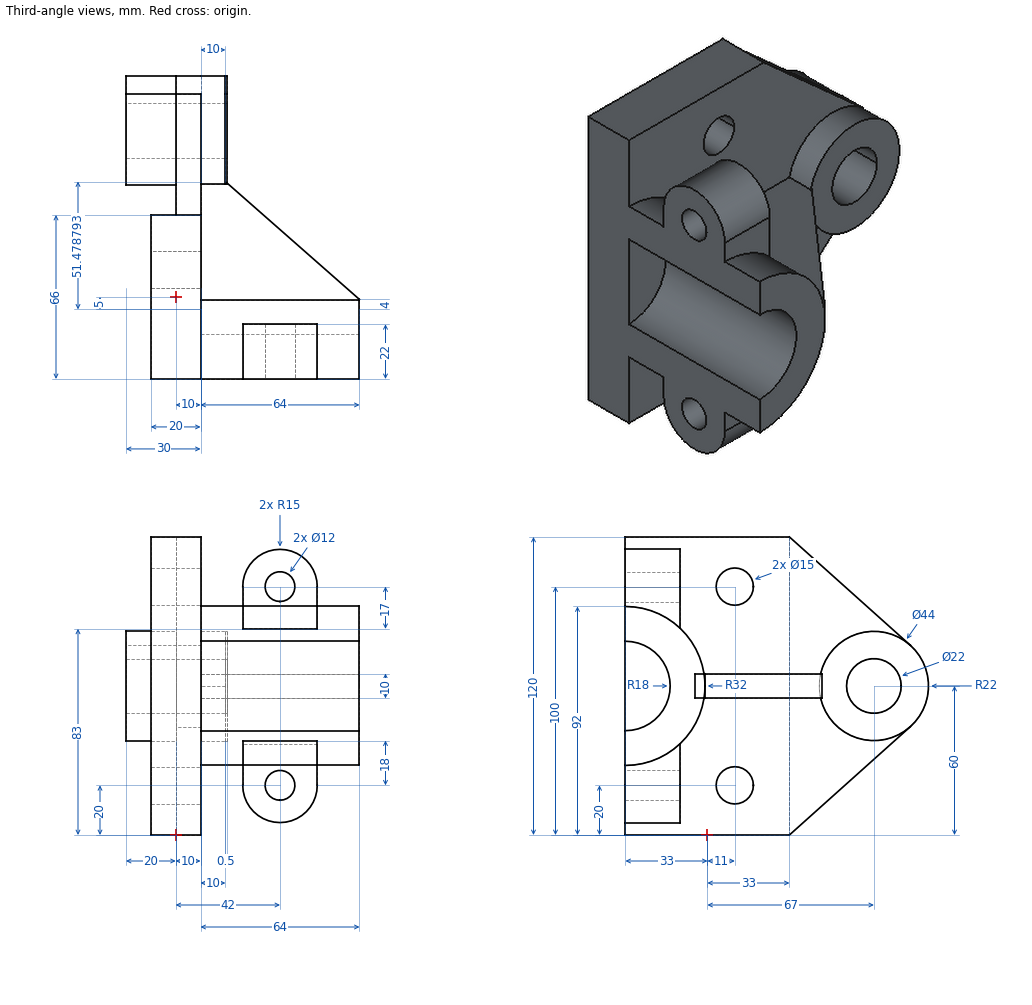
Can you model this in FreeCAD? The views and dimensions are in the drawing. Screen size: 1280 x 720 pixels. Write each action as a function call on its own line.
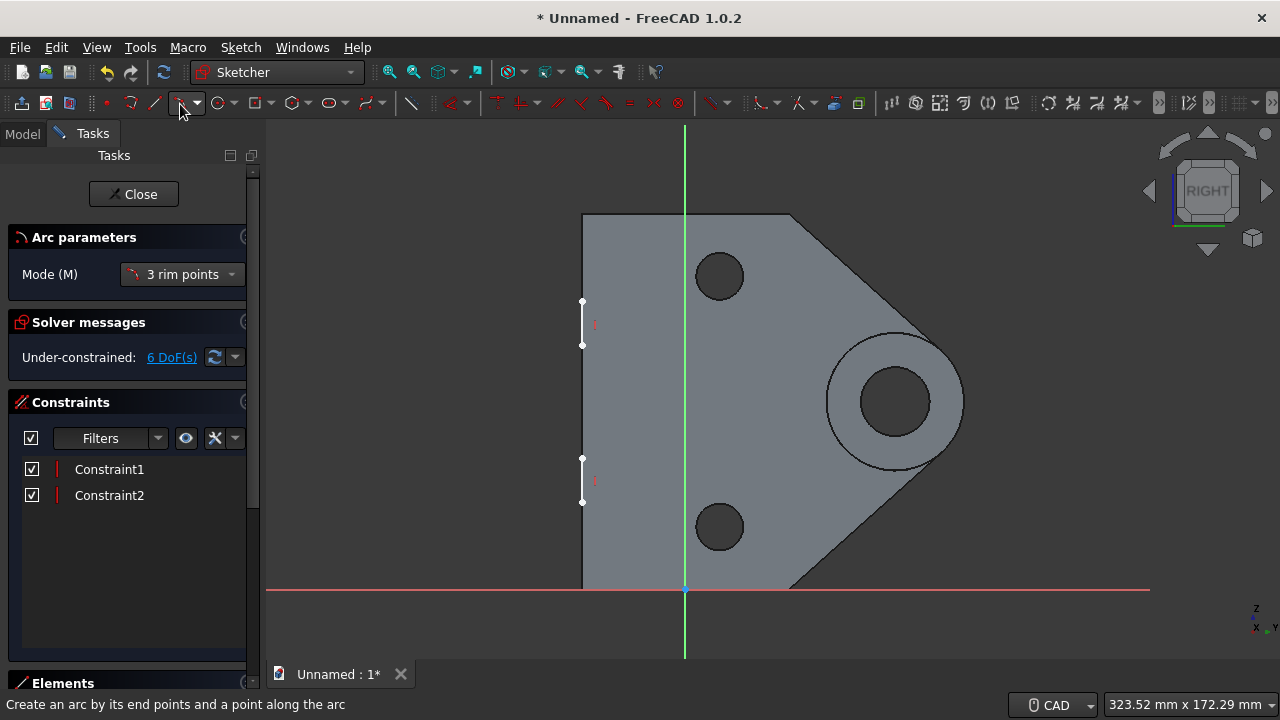
click(582, 346)
click(582, 459)
click(638, 402)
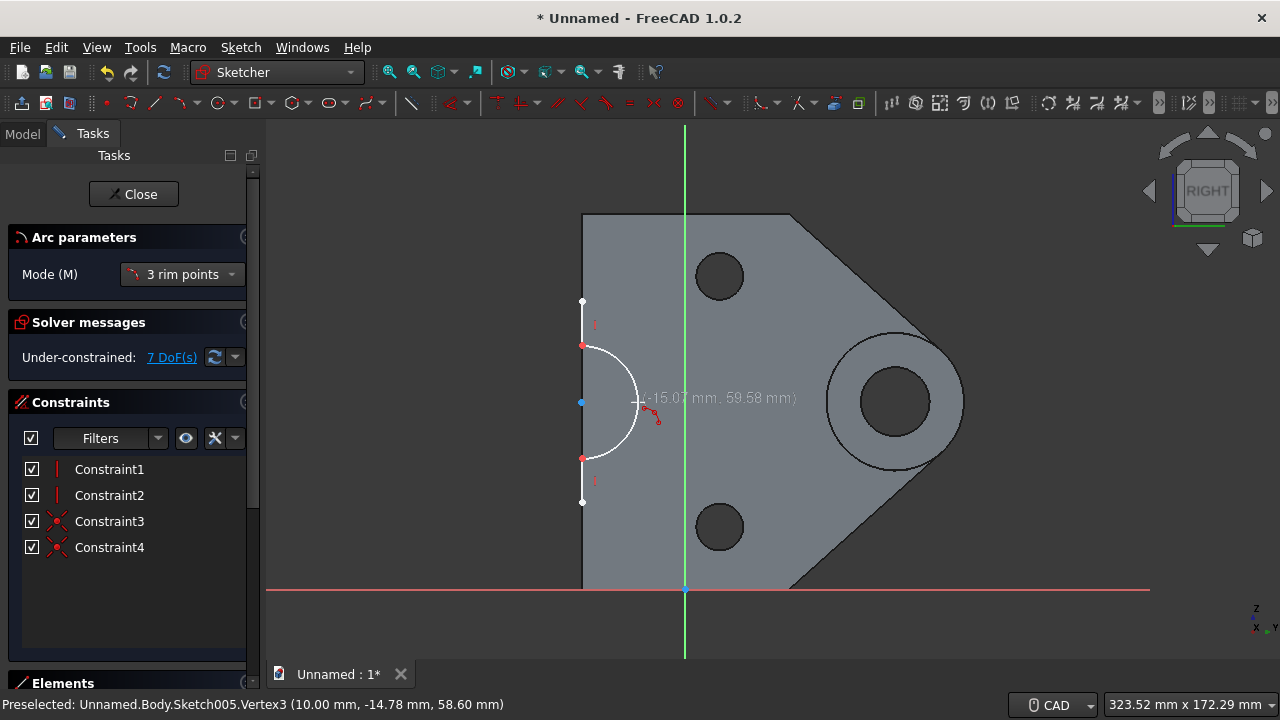
click(582, 503)
click(582, 302)
click(663, 461)
key(Escape)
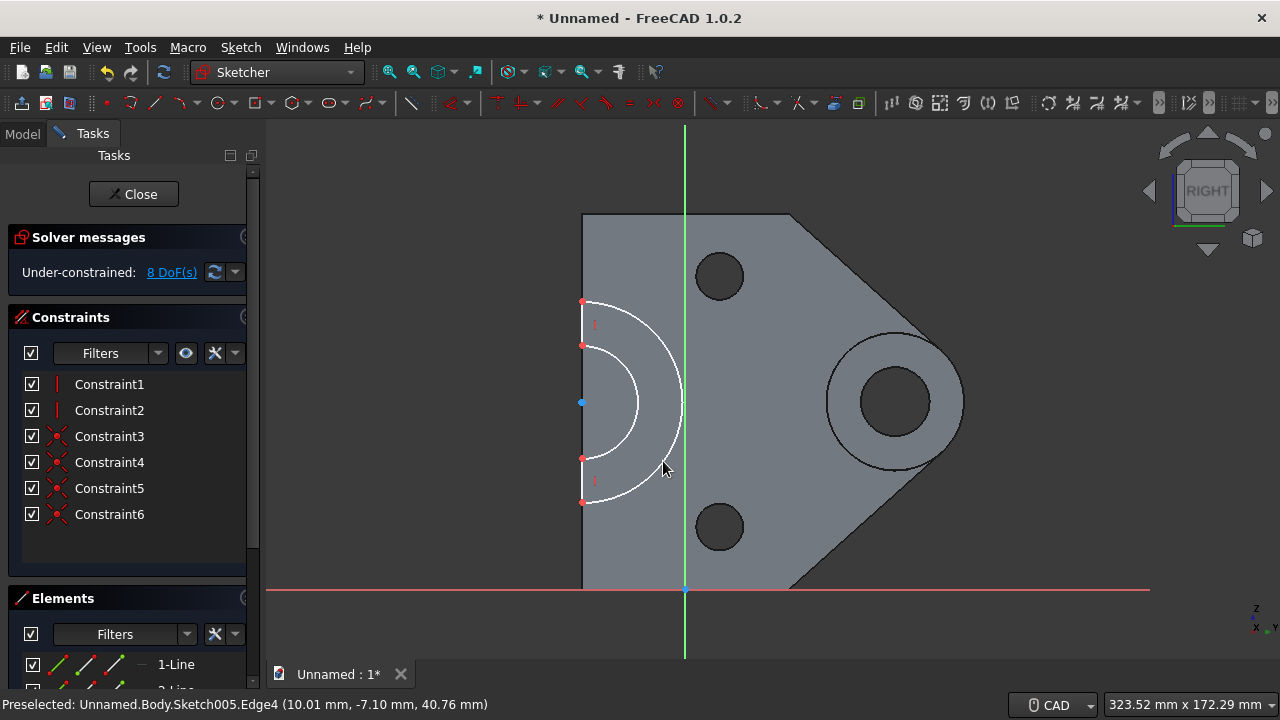
click(627, 436)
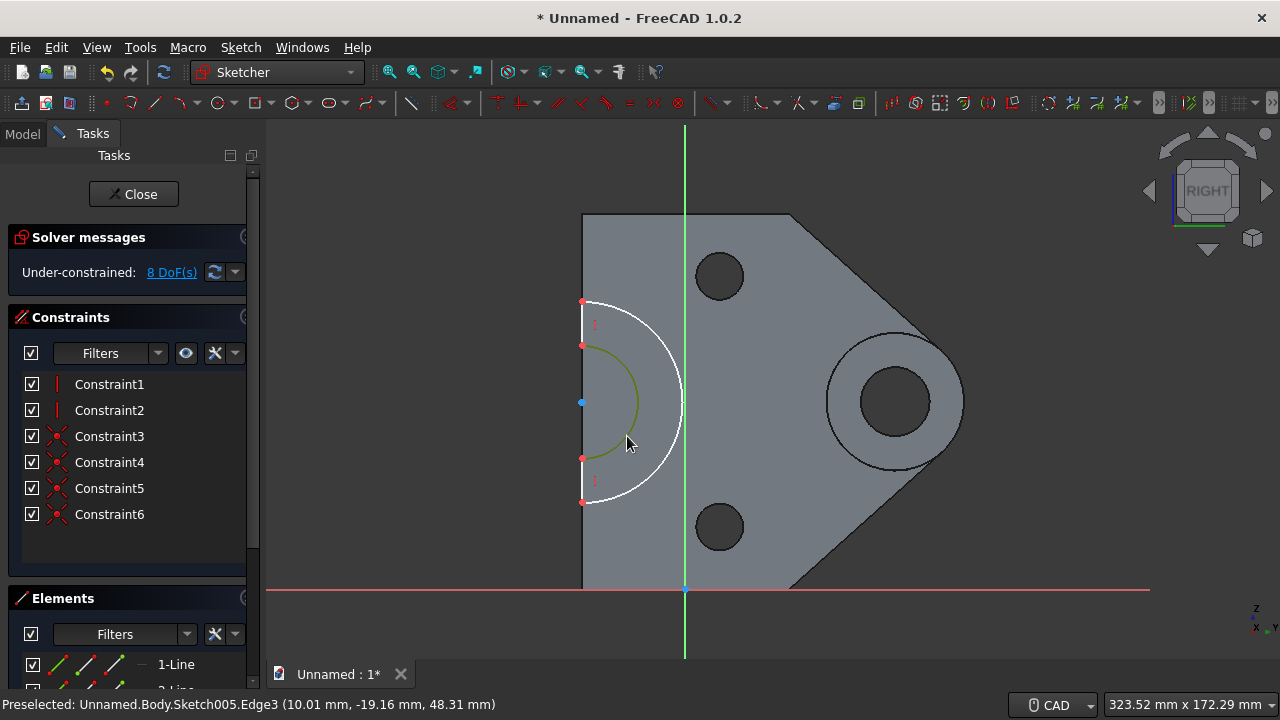
click(663, 462)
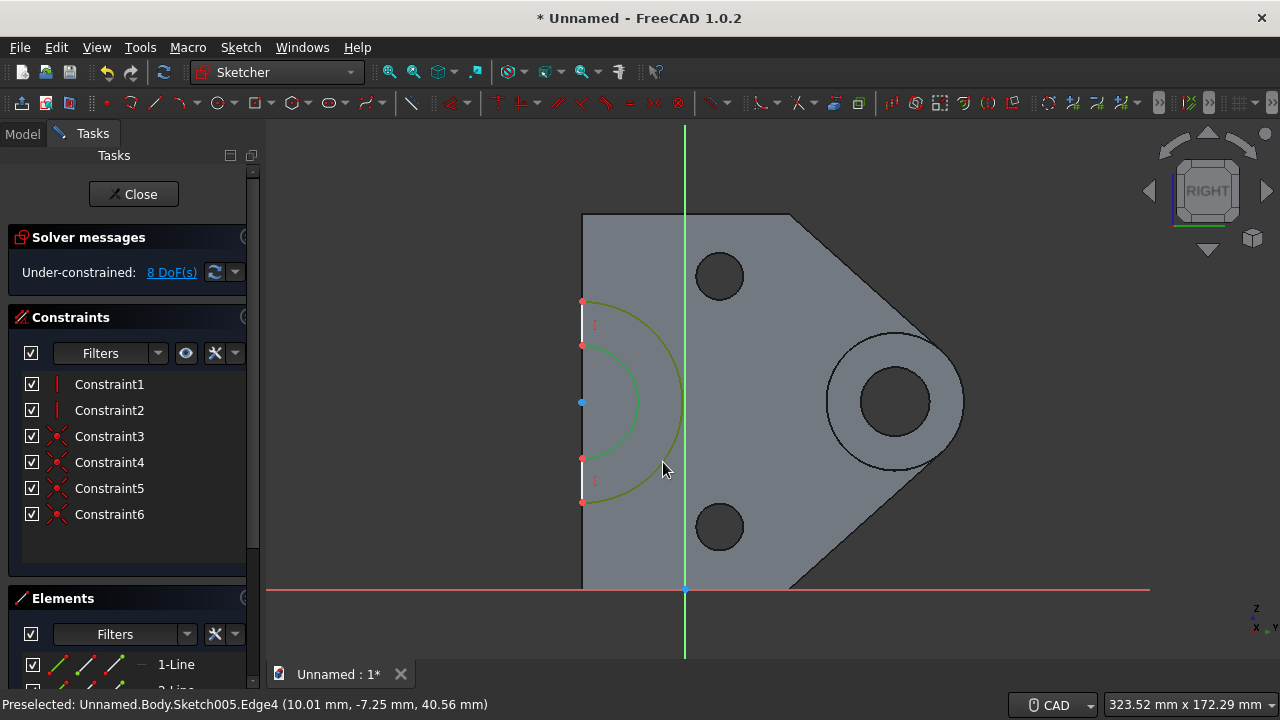
click(498, 104)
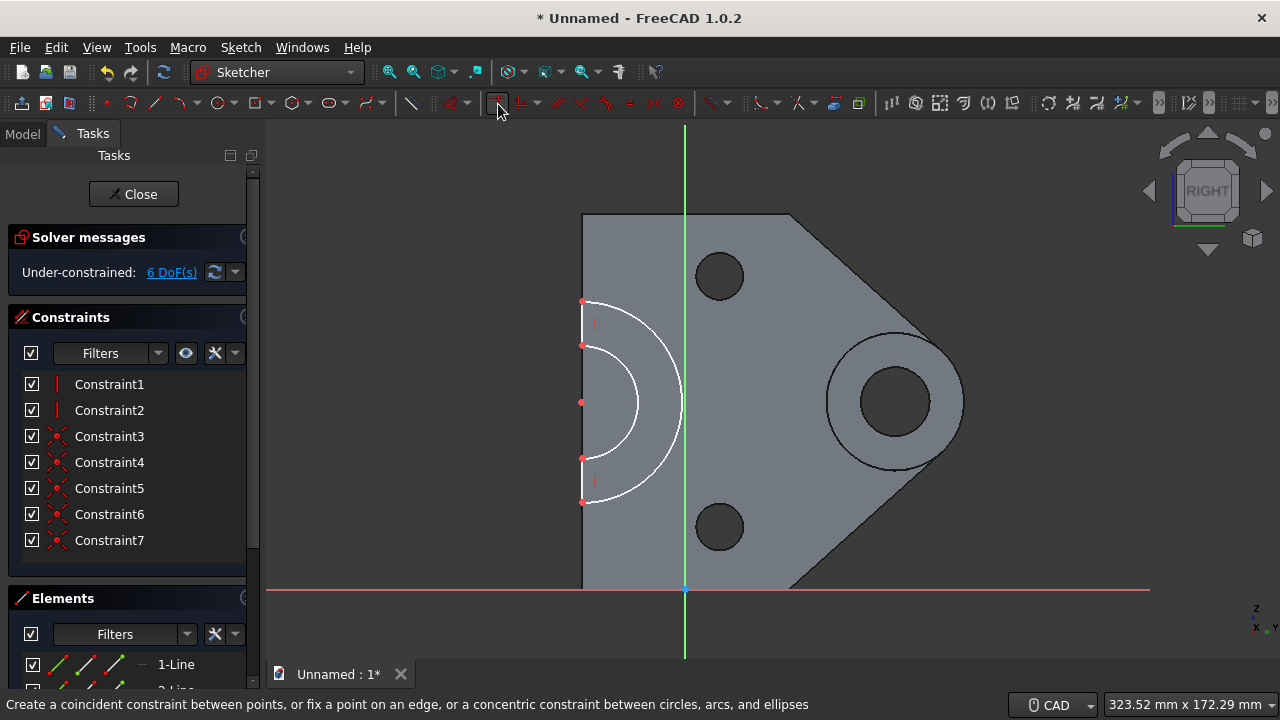
click(450, 104)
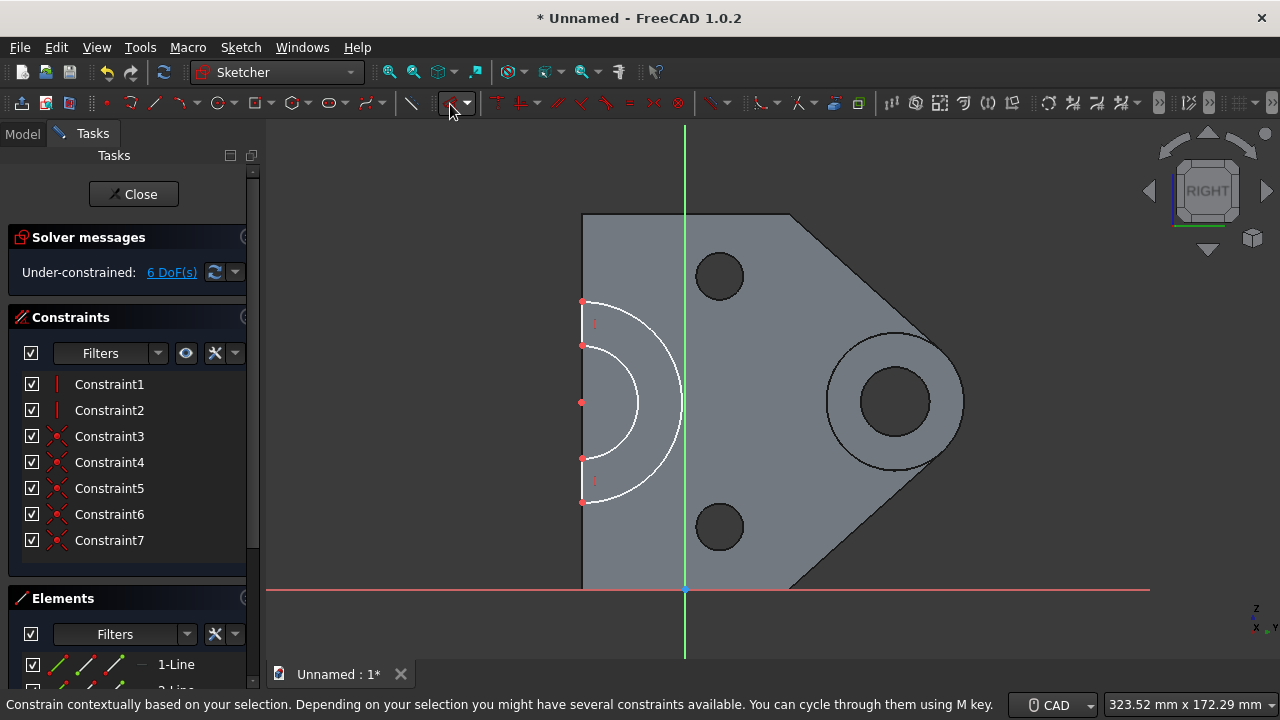
click(627, 436)
click(529, 474)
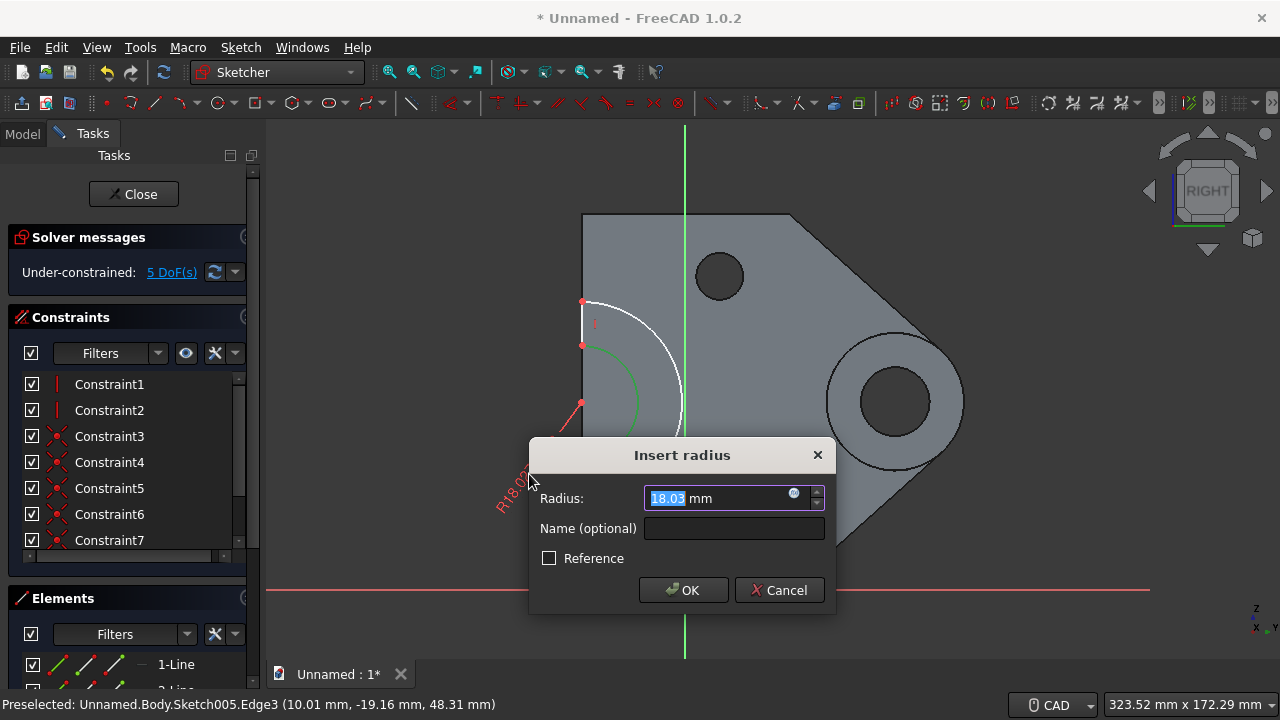
text(18)
key(Return)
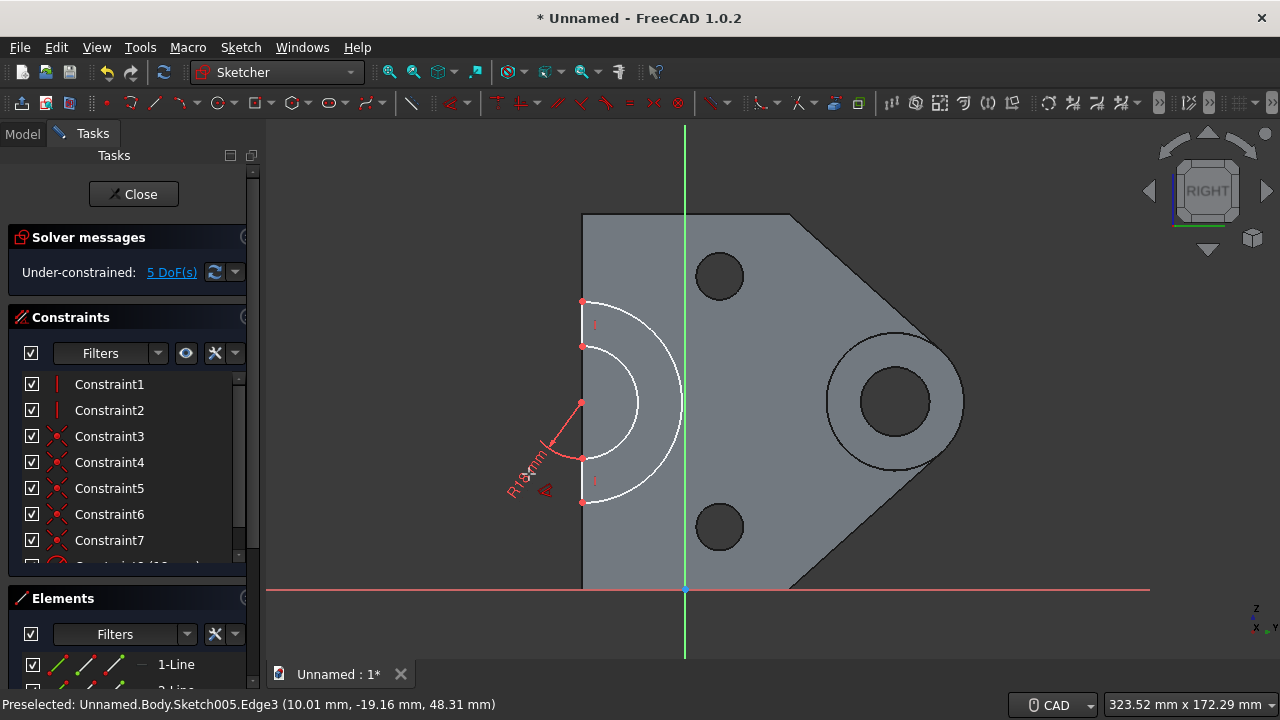
click(663, 461)
click(639, 522)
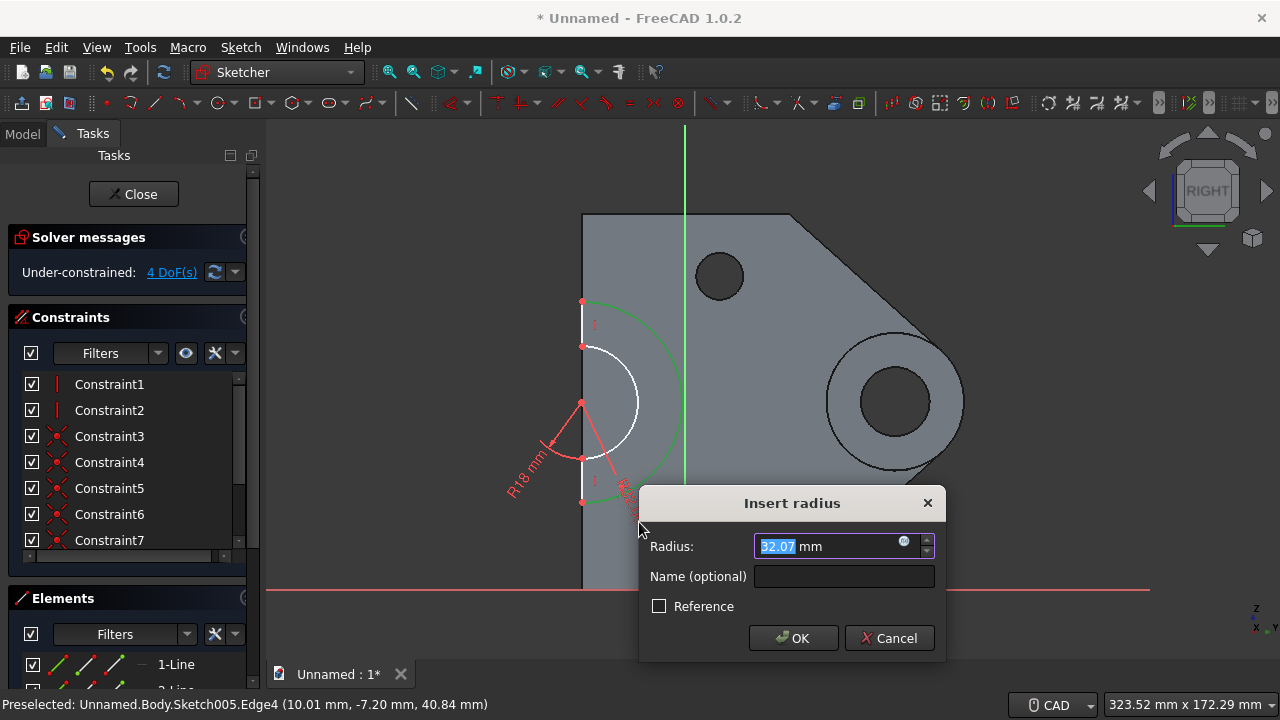
text(32)
key(Return)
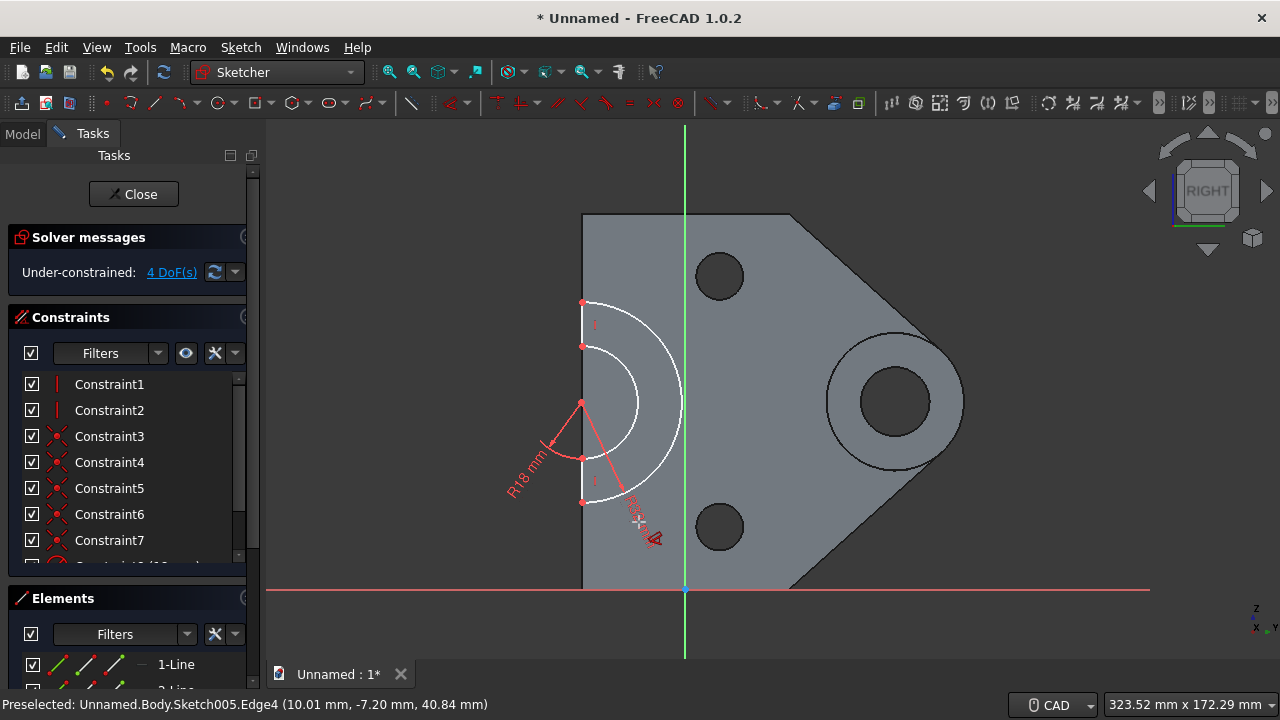
click(582, 302)
click(634, 624)